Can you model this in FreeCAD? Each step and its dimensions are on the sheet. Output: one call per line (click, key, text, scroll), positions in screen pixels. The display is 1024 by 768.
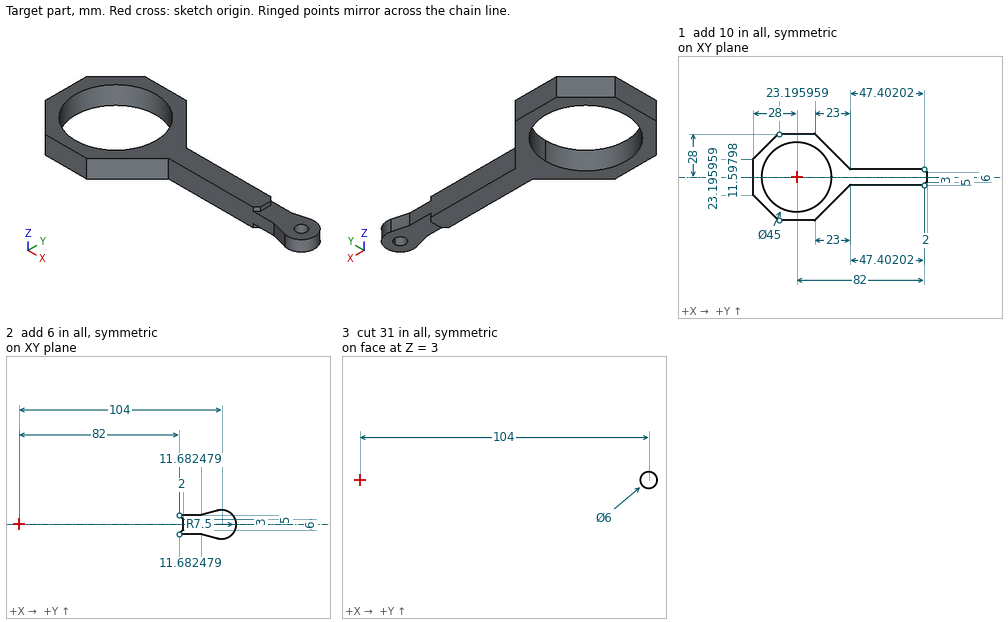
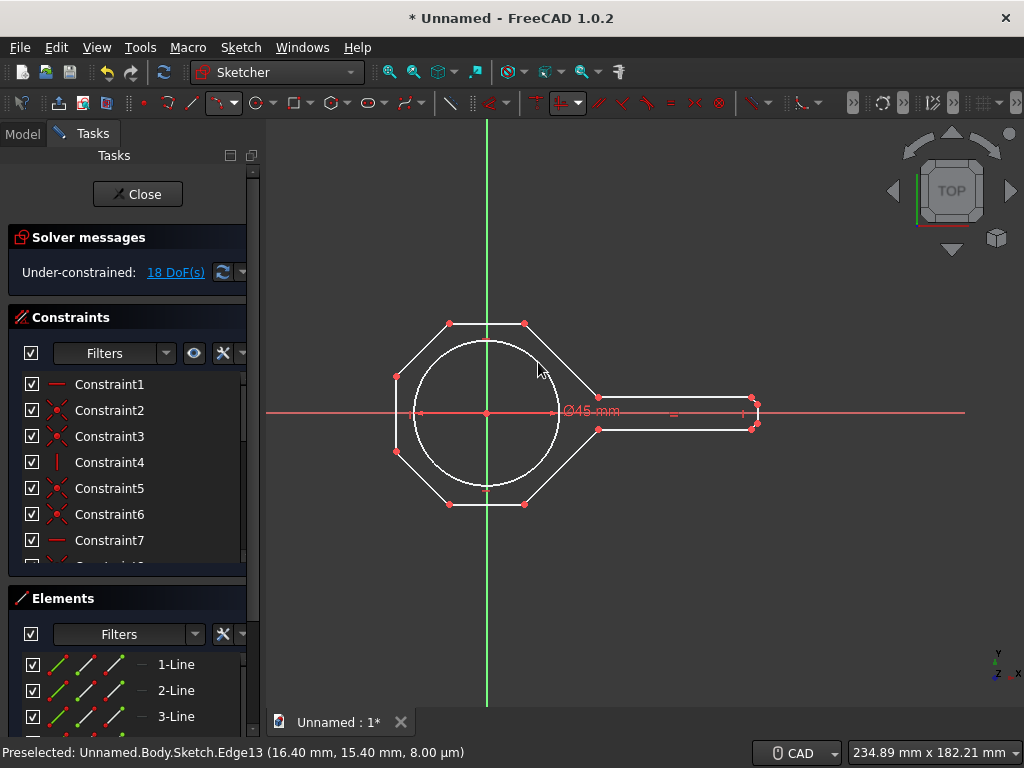
click(449, 324)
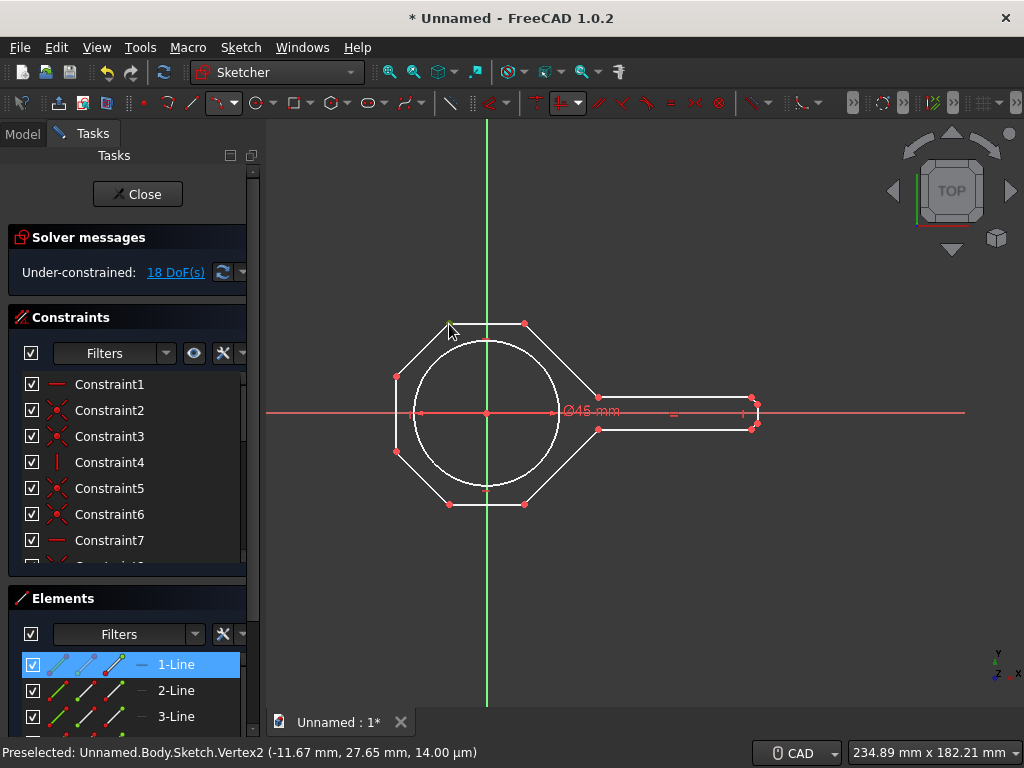
click(449, 505)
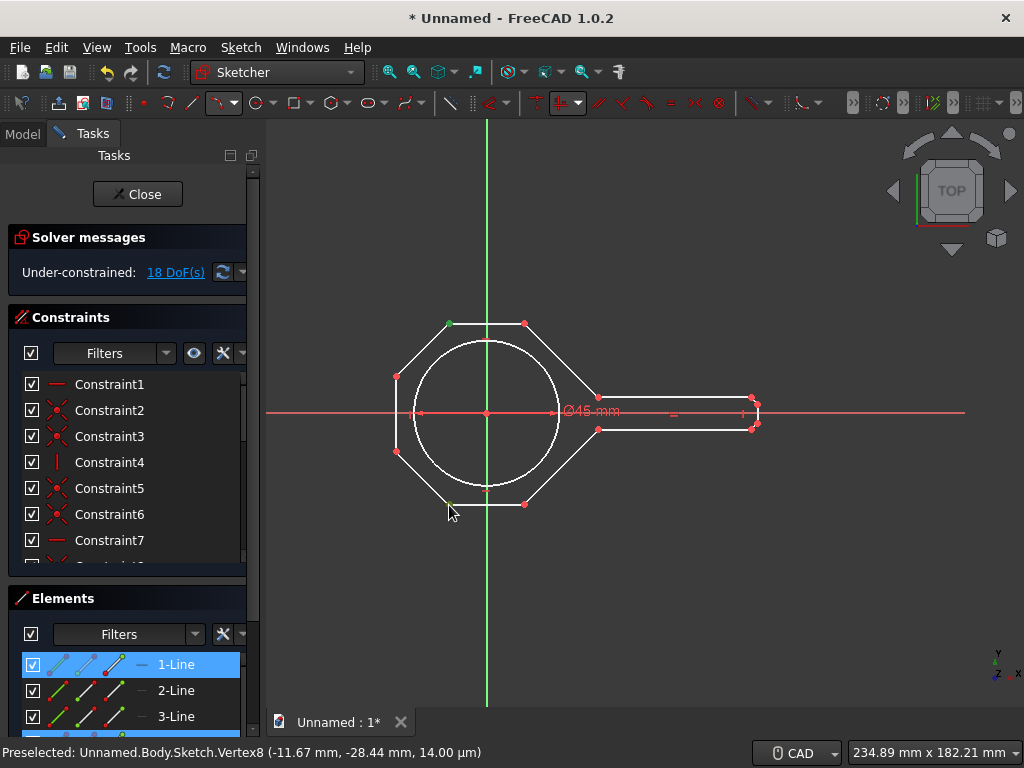
click(334, 413)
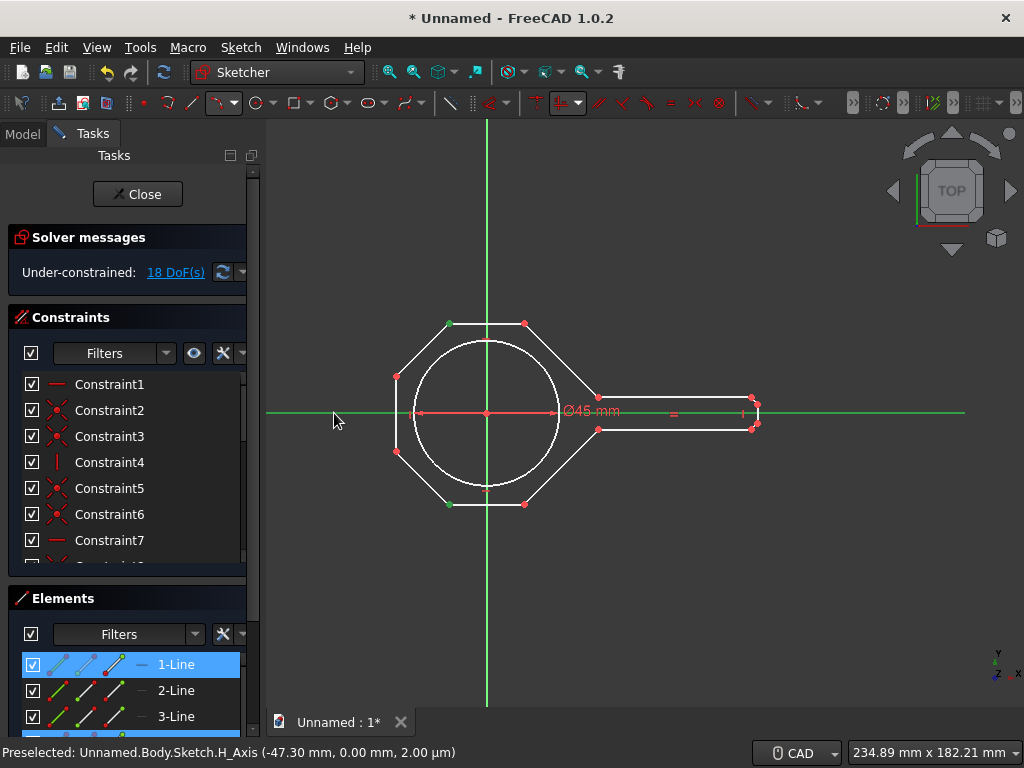
click(696, 104)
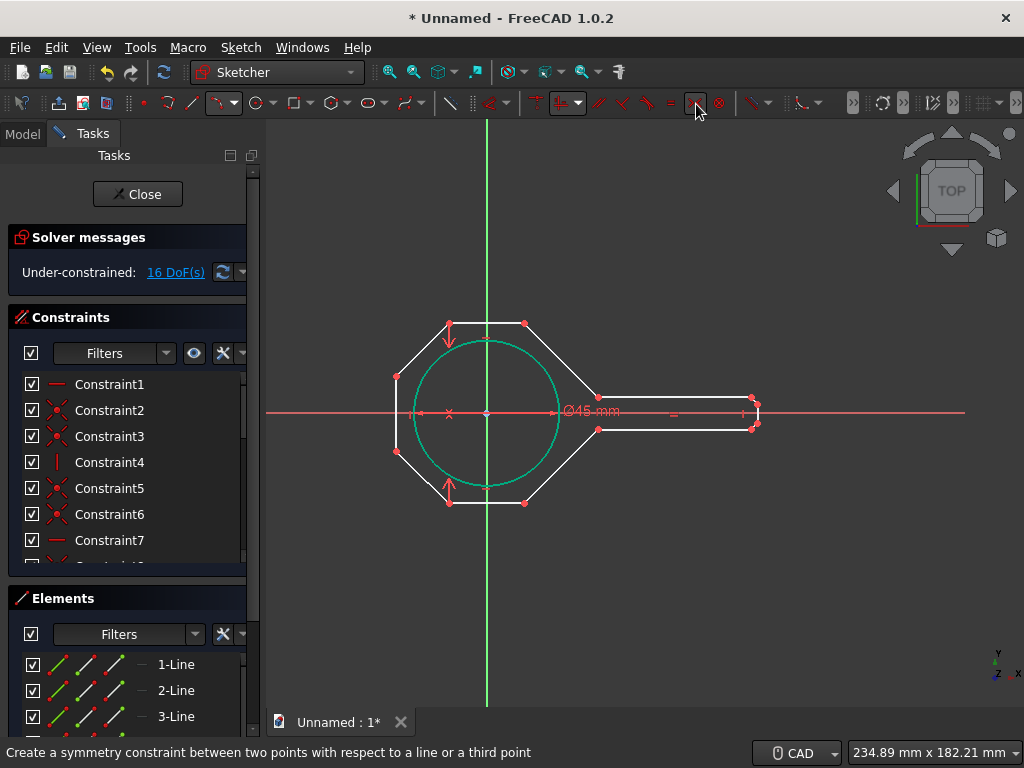
scroll(751, 430, up, 2)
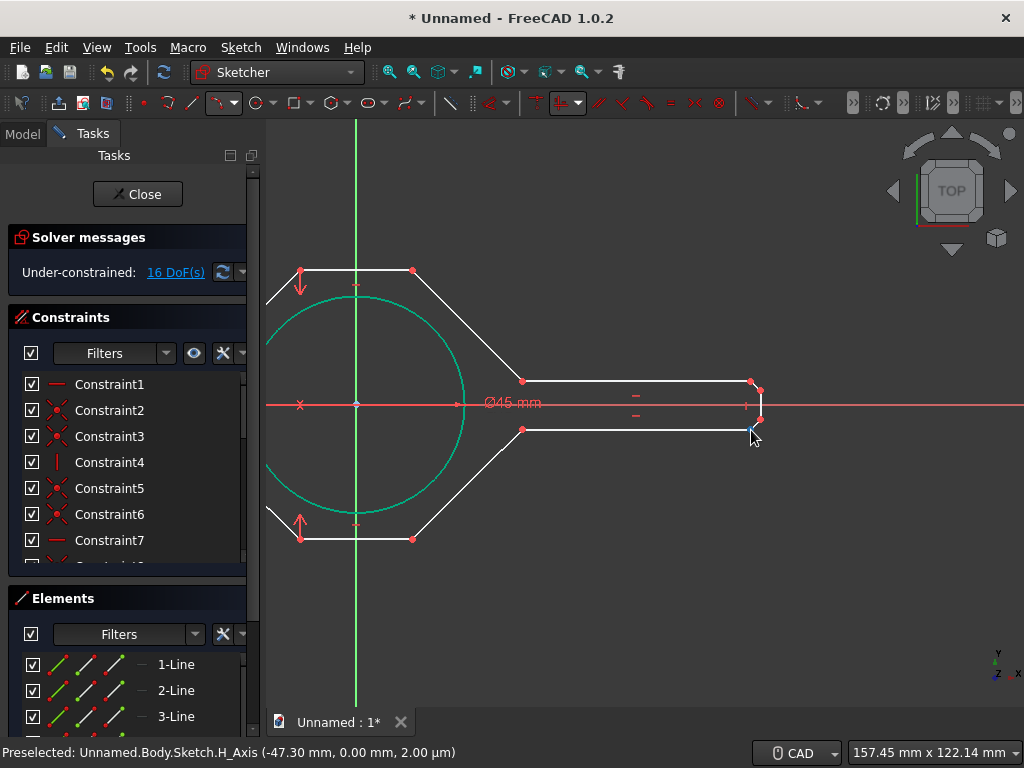
click(751, 430)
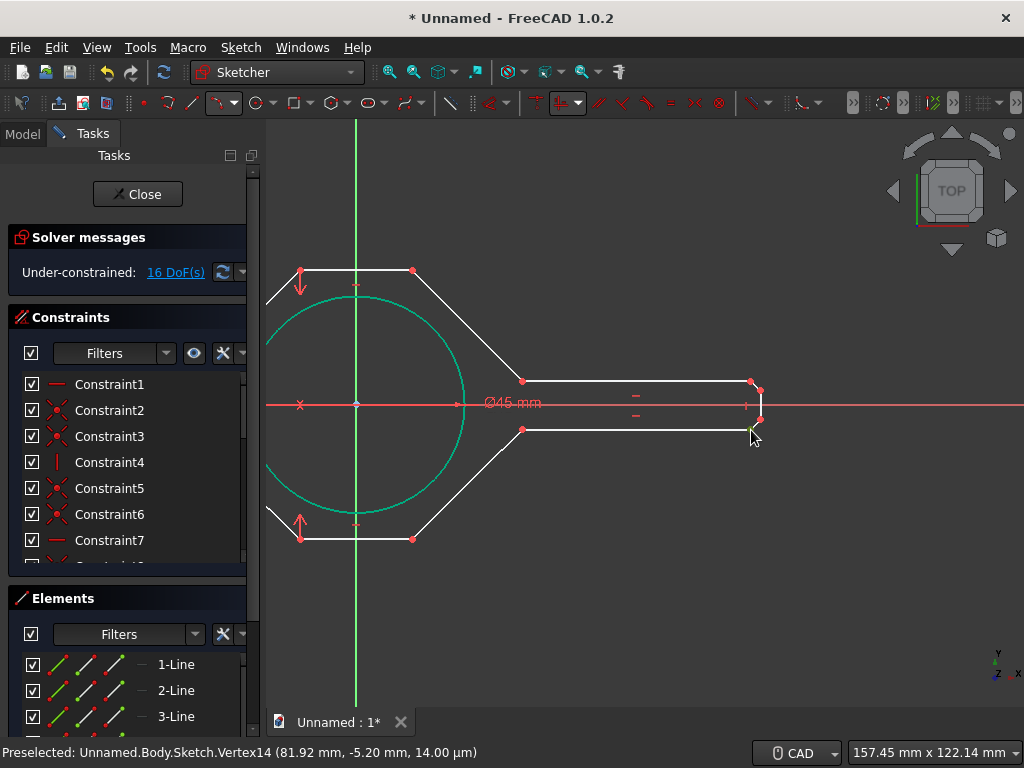
click(751, 381)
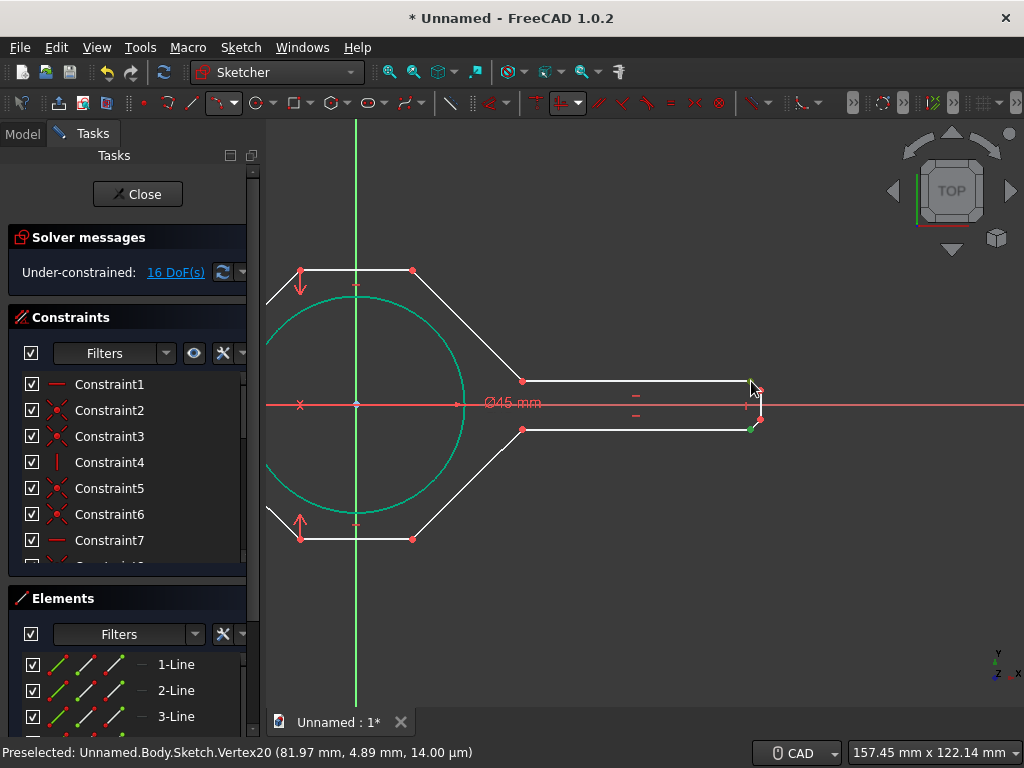
click(415, 405)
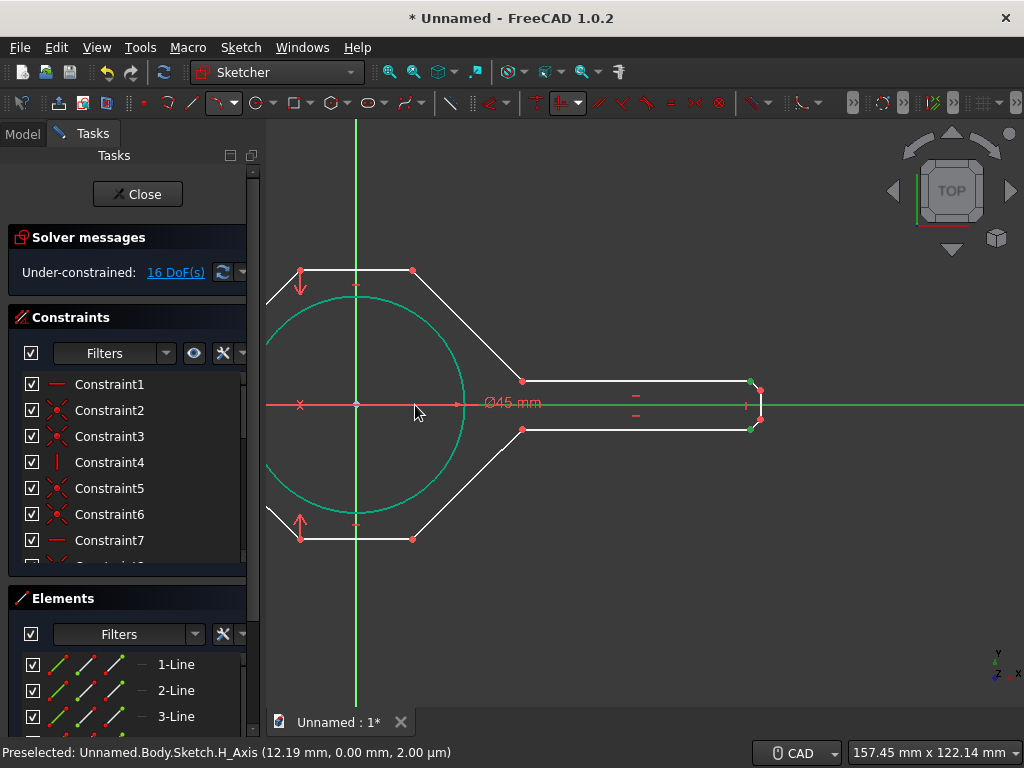
click(696, 104)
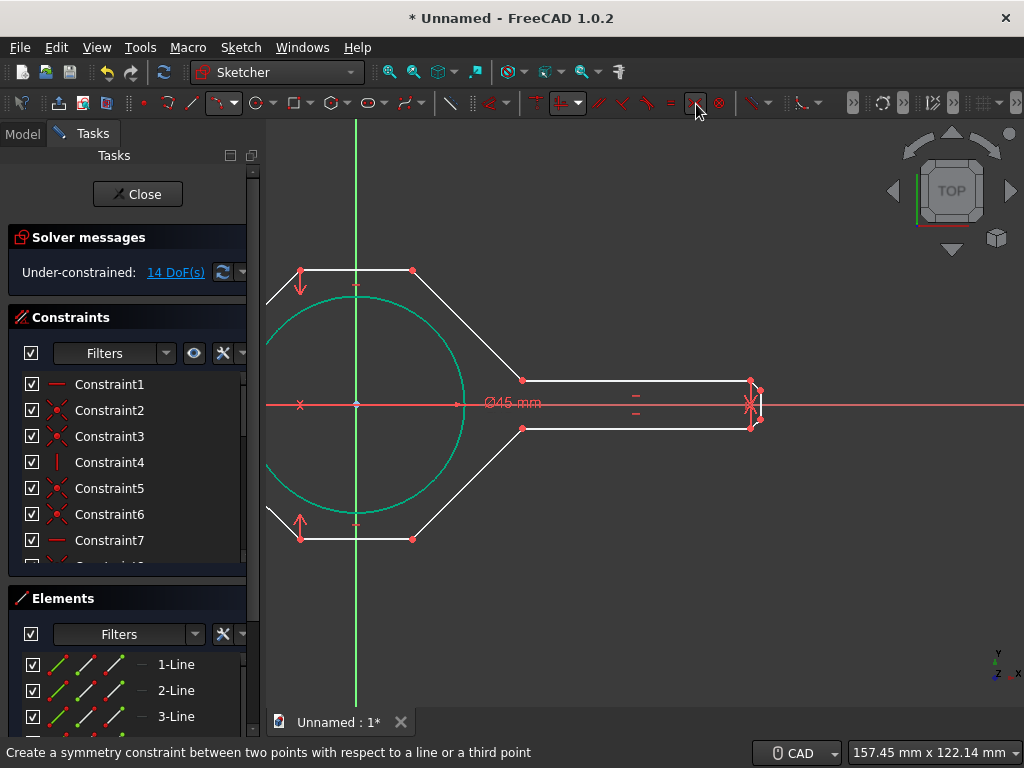
scroll(761, 408, up, 2)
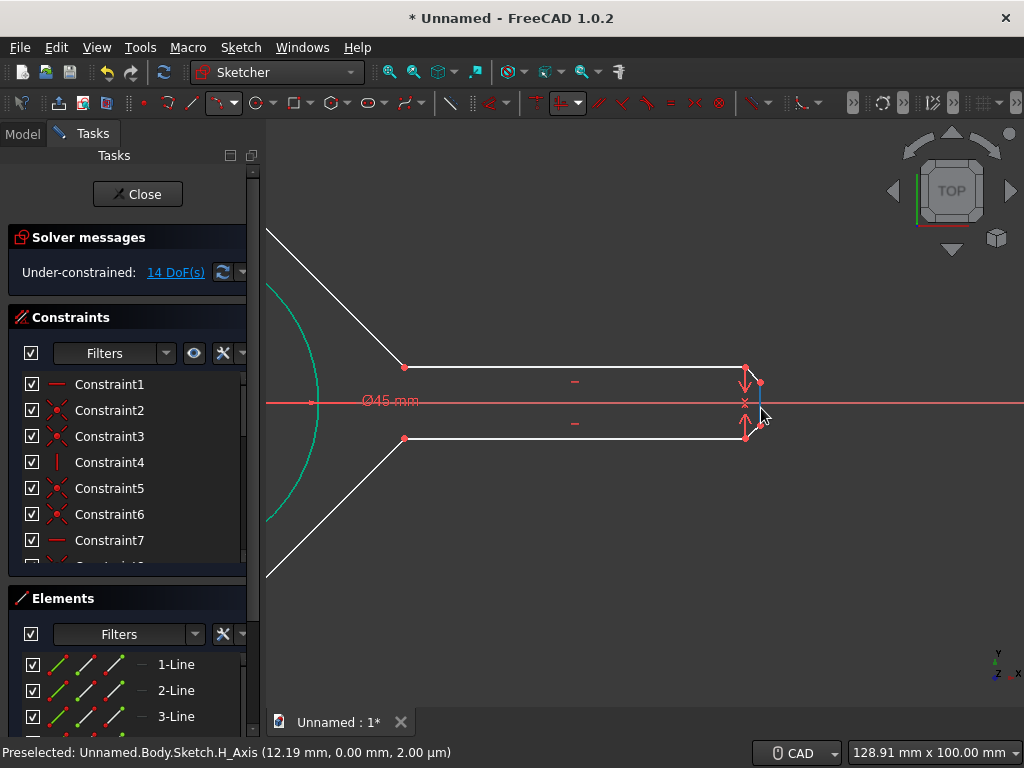
click(760, 408)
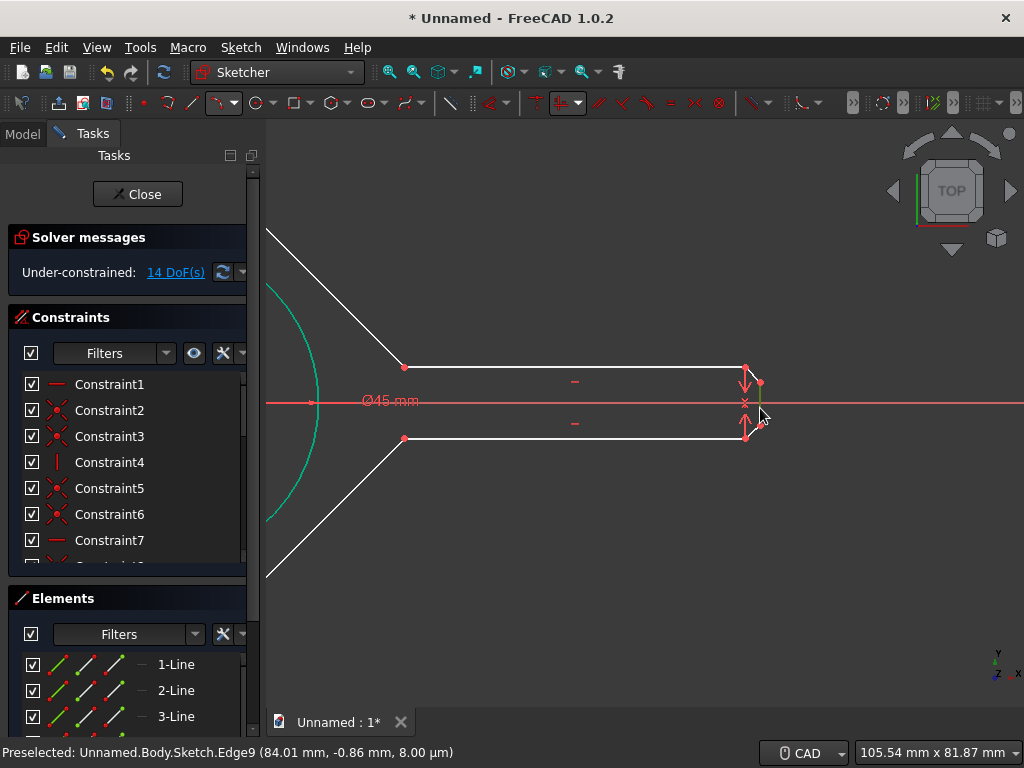
key(i)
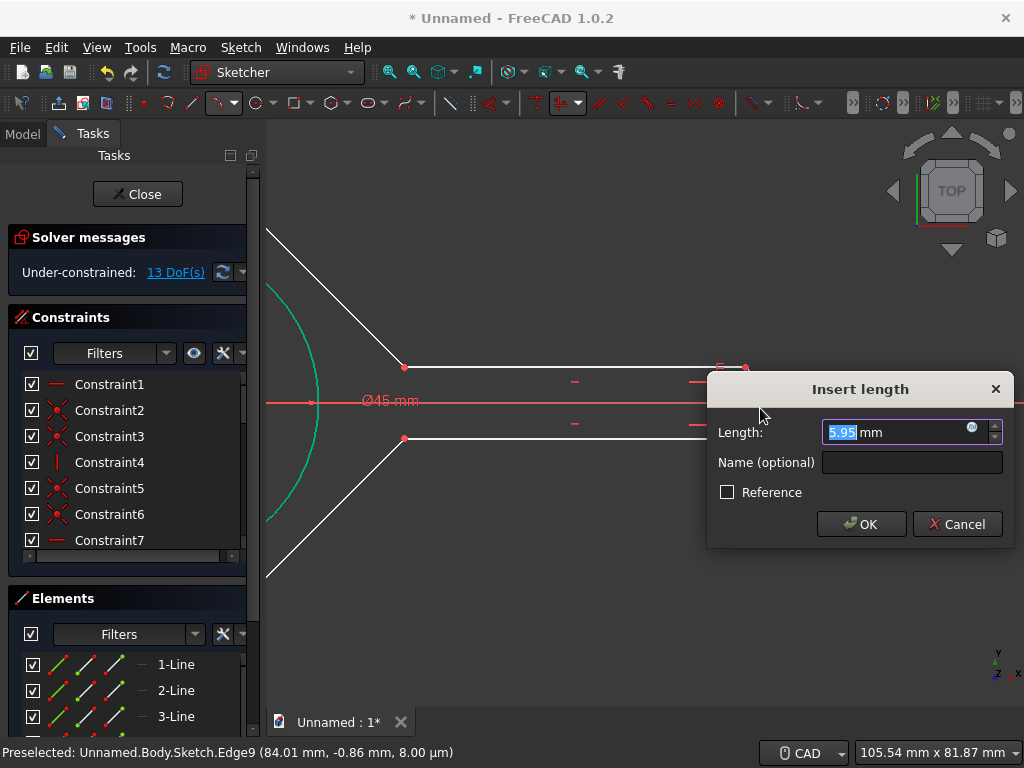
text(6)
key(Return)